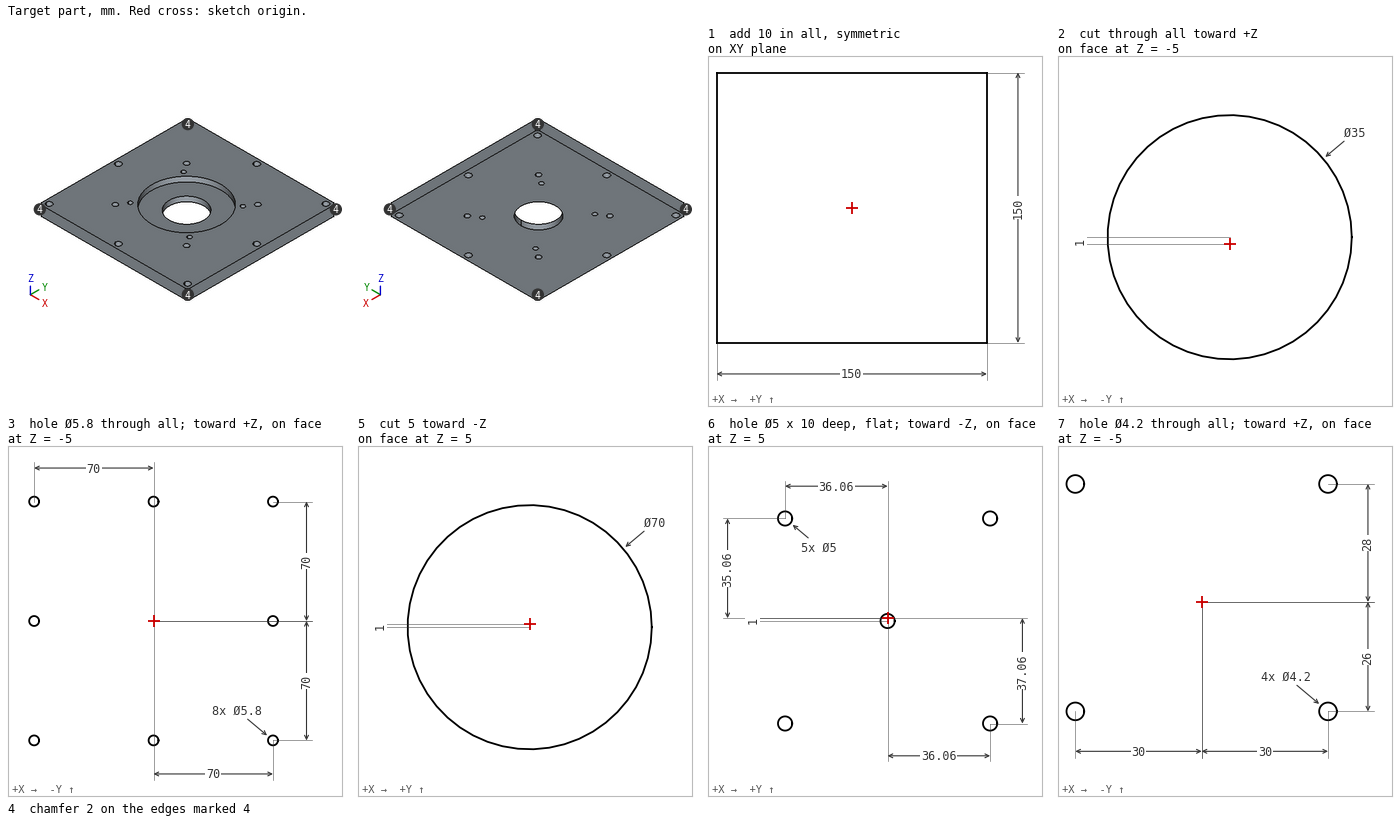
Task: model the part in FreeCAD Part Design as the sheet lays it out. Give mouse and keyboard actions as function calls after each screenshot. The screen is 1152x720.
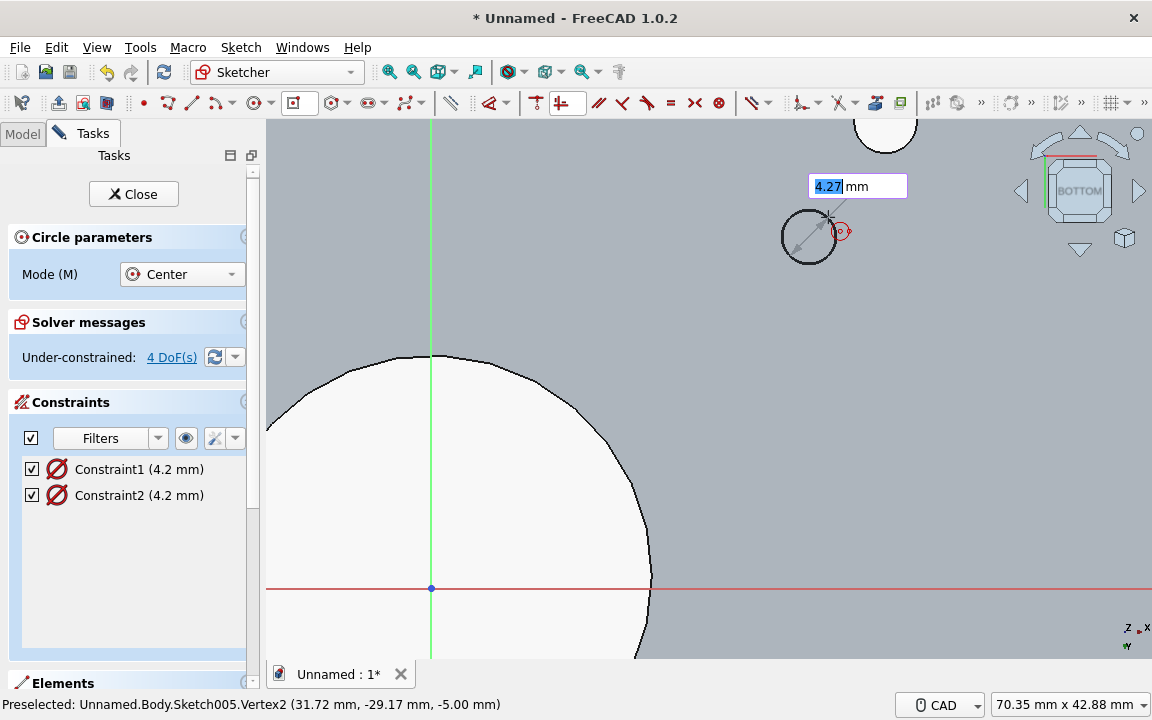
text(4.2)
key(Return)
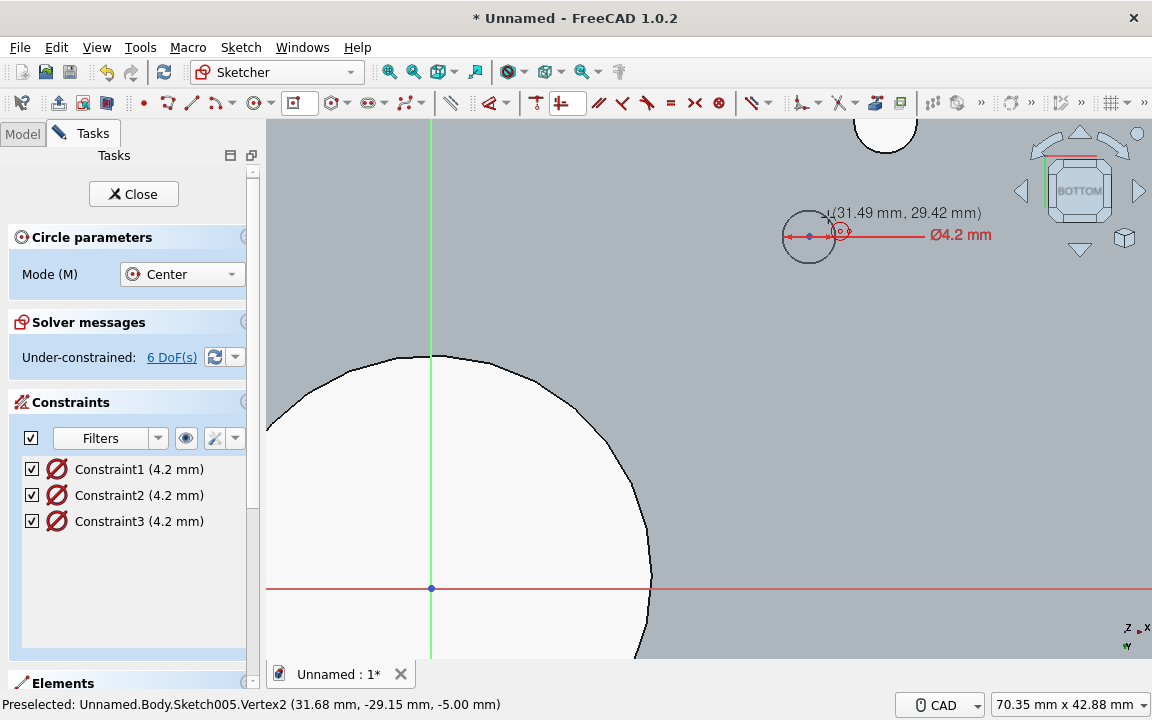
scroll(811, 236, down, 4)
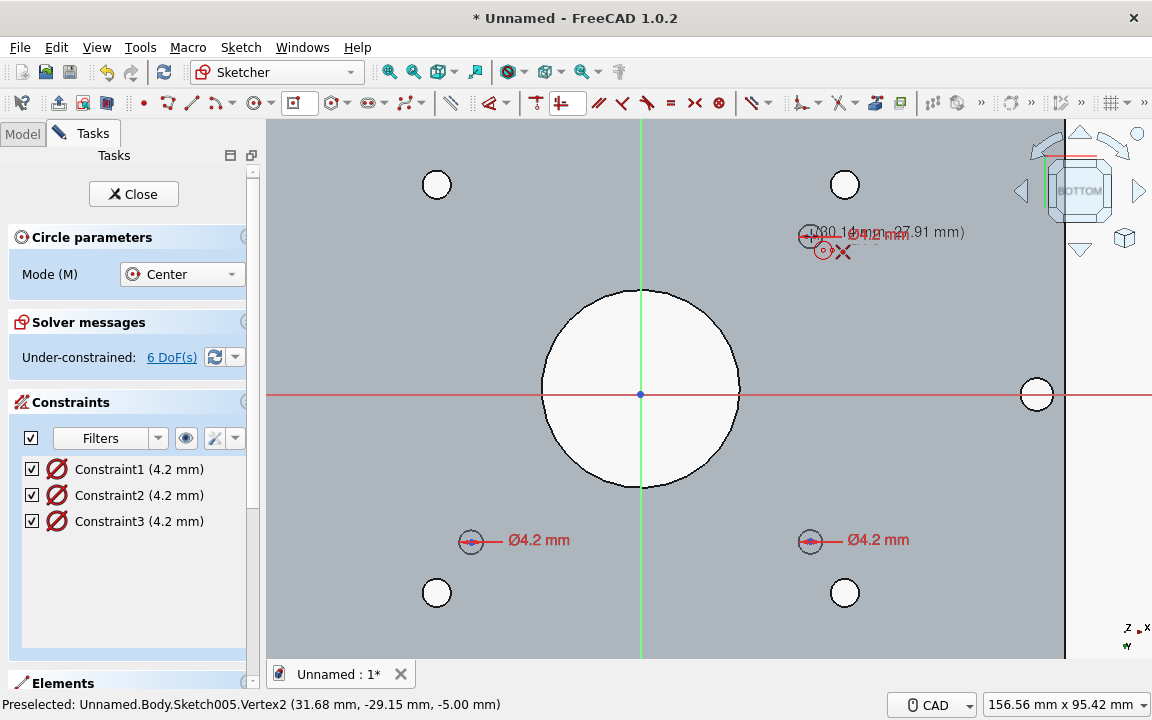
scroll(471, 236, up, 4)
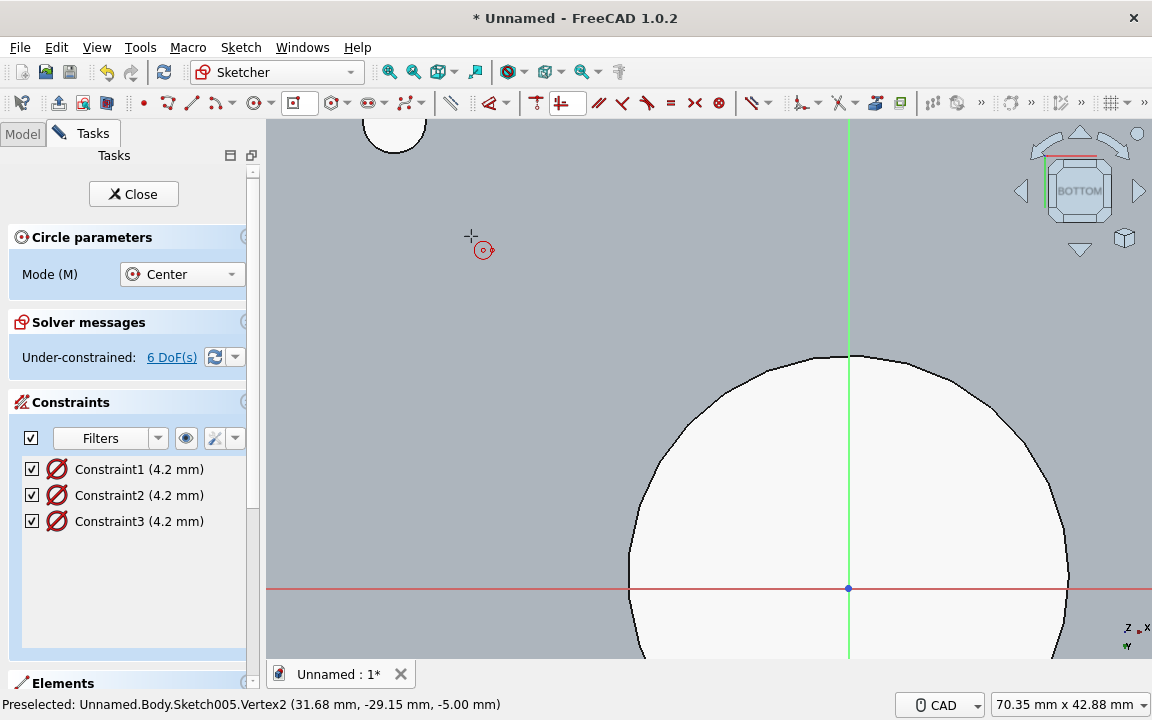
click(471, 236)
move(489, 217)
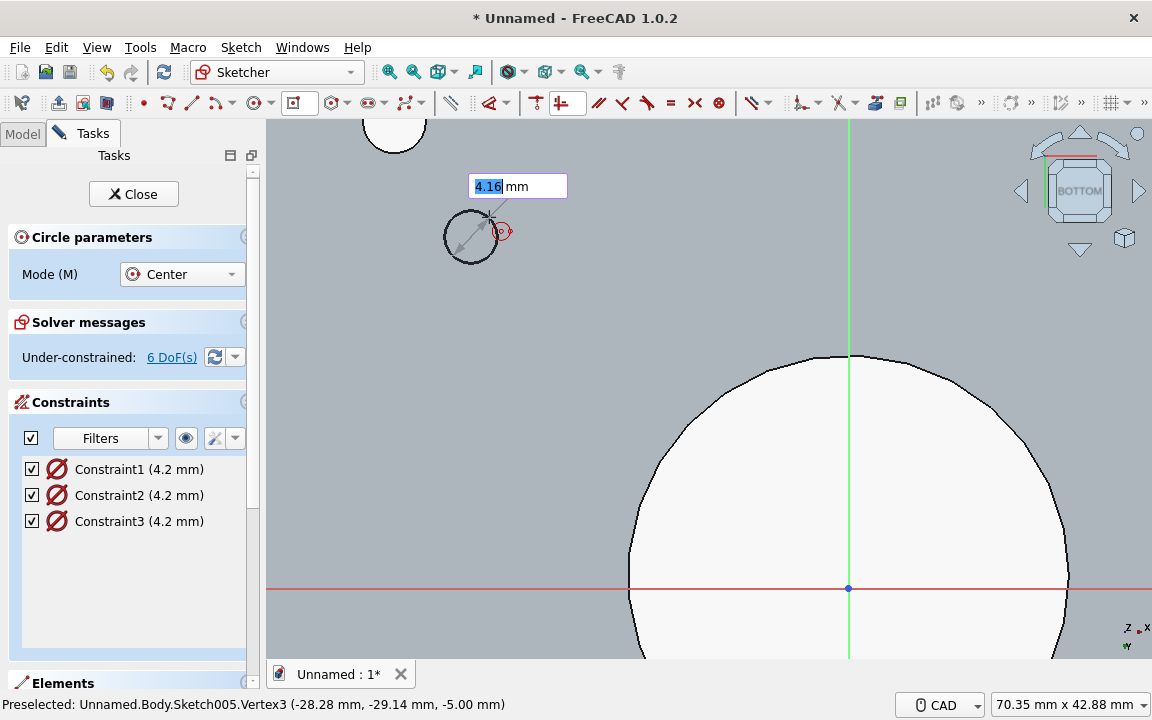
text(4.2)
key(Return)
key(Escape)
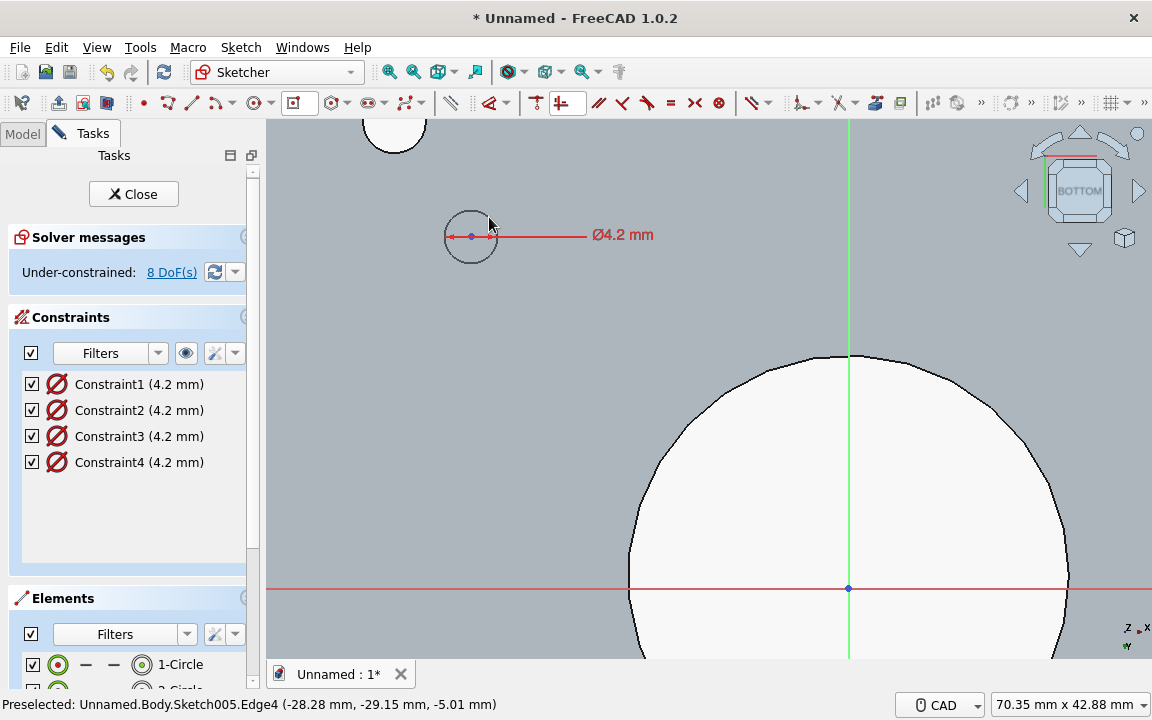
scroll(471, 236, down, 4)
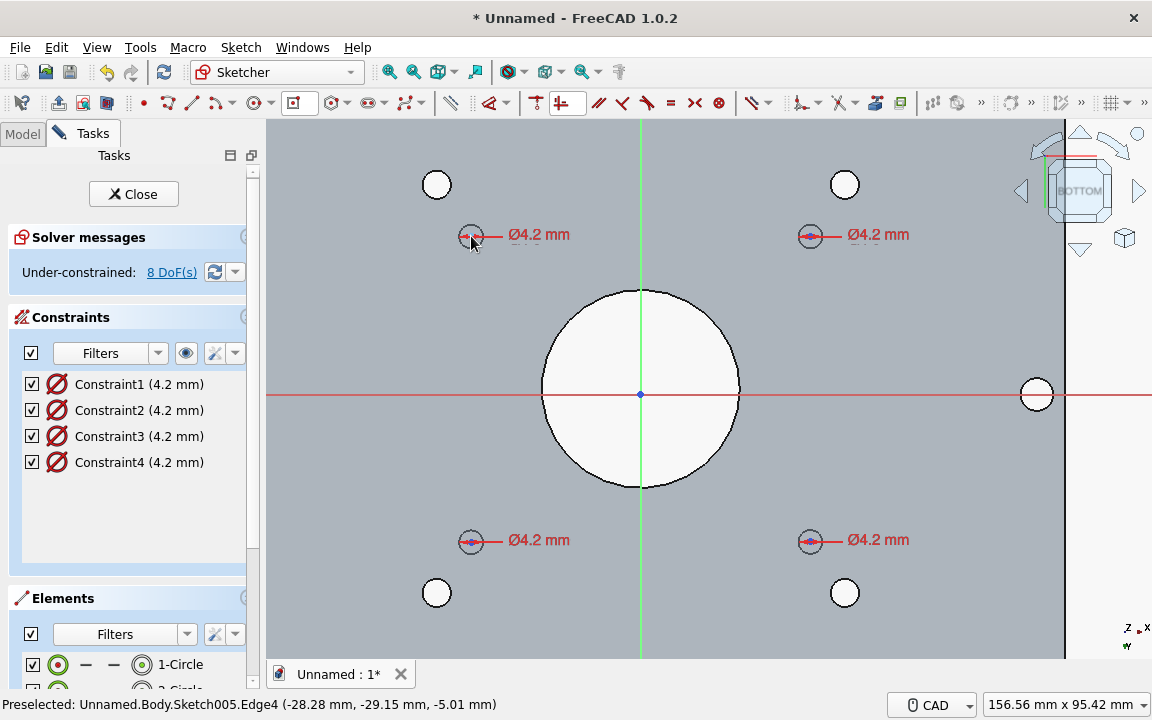
click(810, 542)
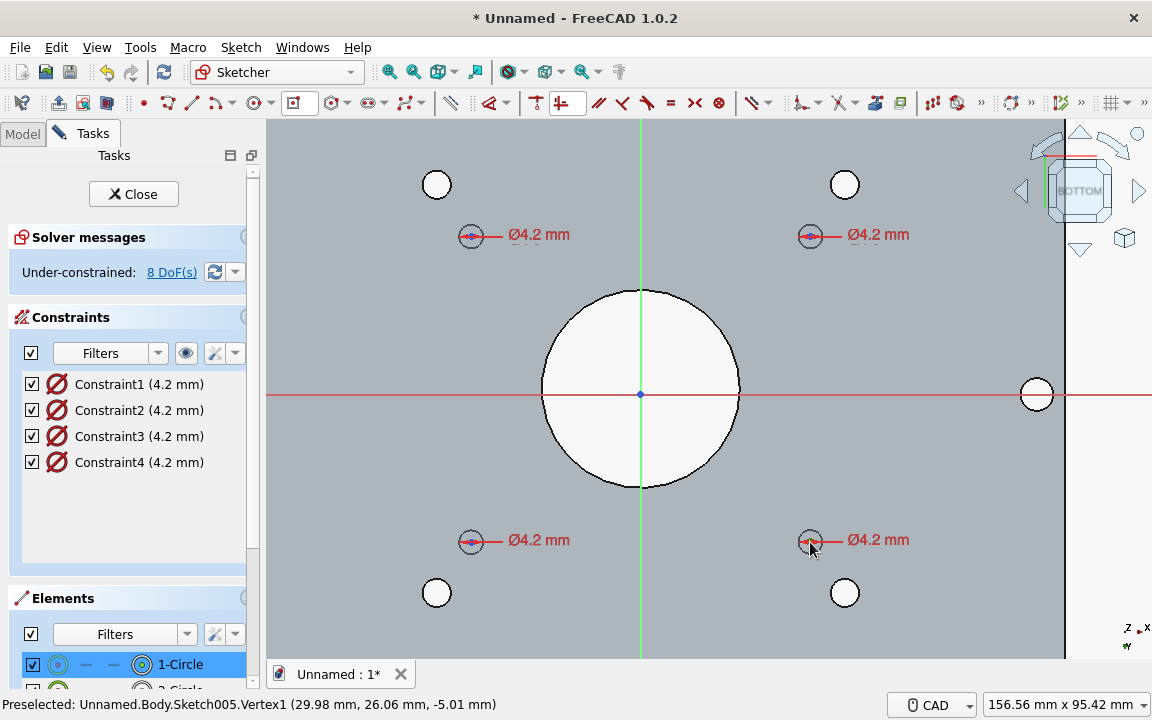
click(471, 542)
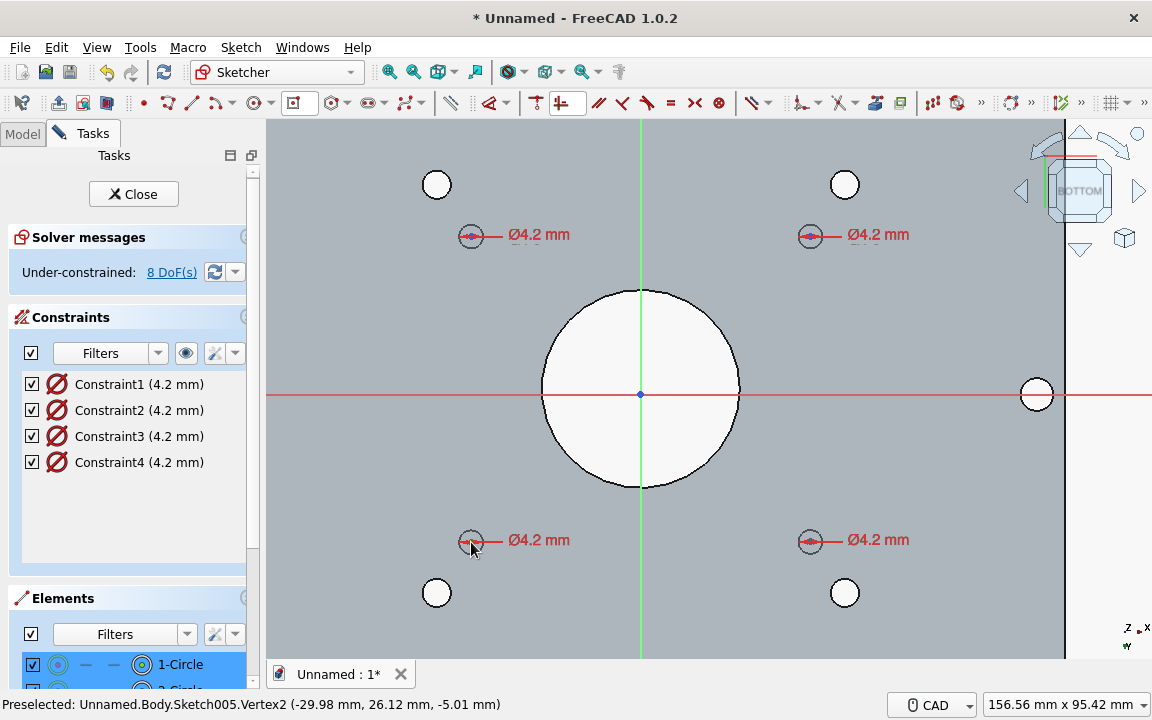
key(h)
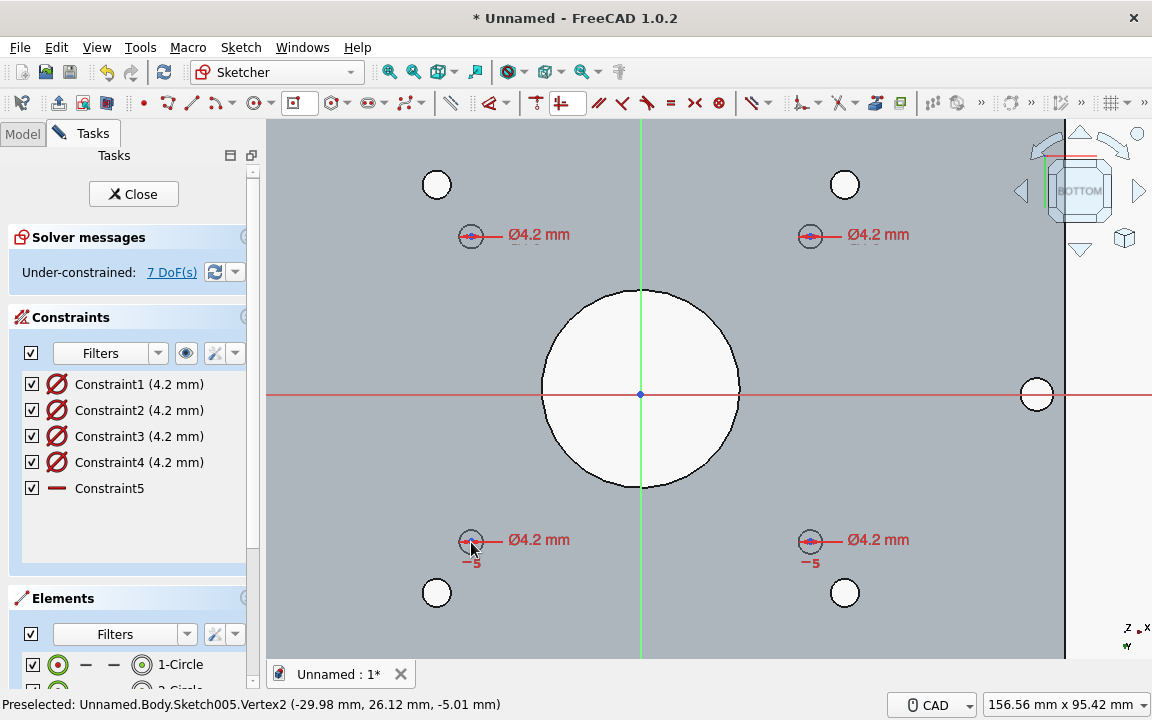
click(810, 542)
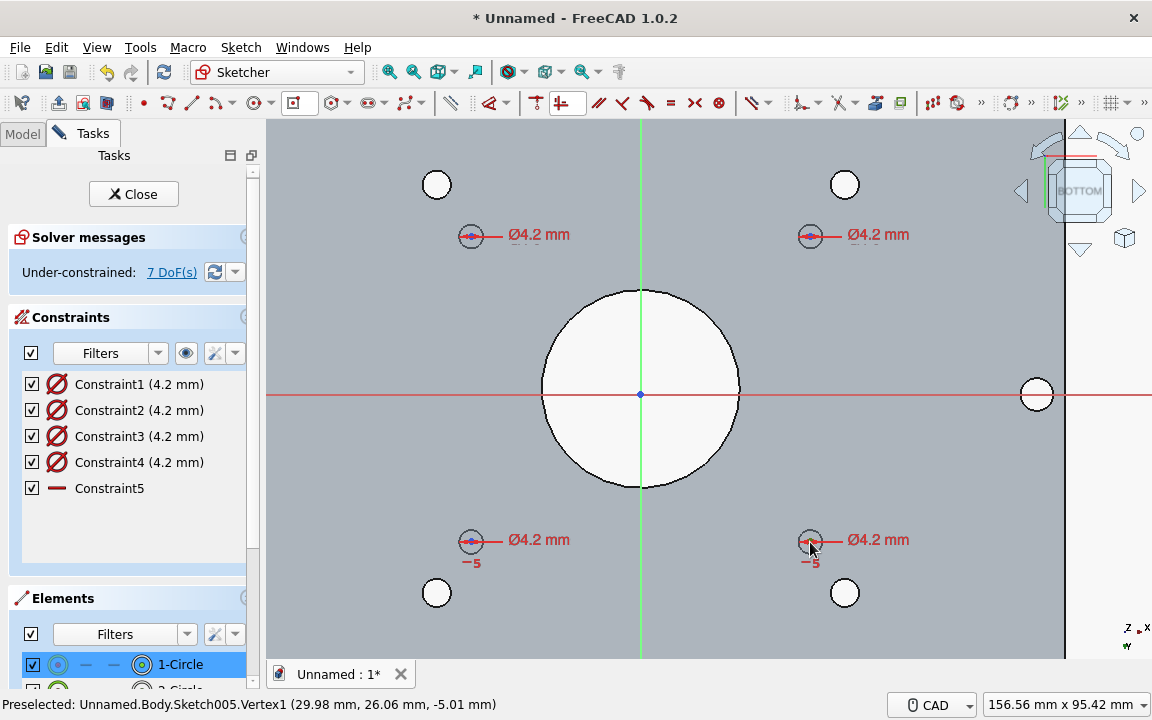
click(810, 237)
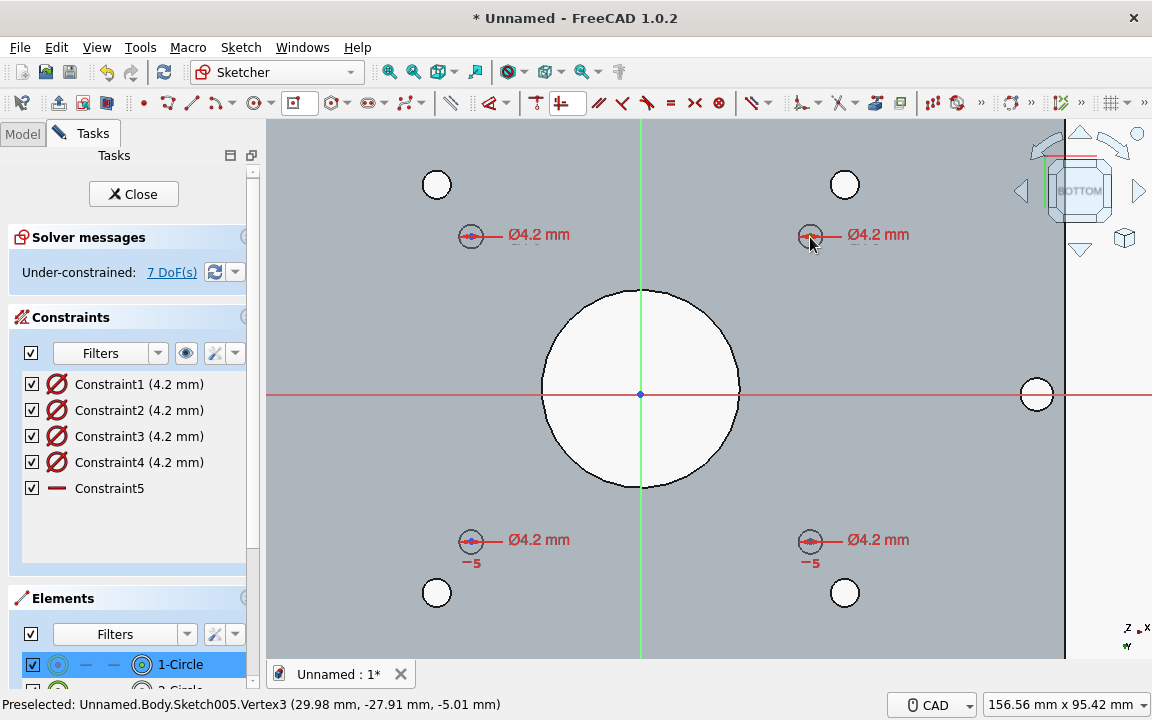
key(v)